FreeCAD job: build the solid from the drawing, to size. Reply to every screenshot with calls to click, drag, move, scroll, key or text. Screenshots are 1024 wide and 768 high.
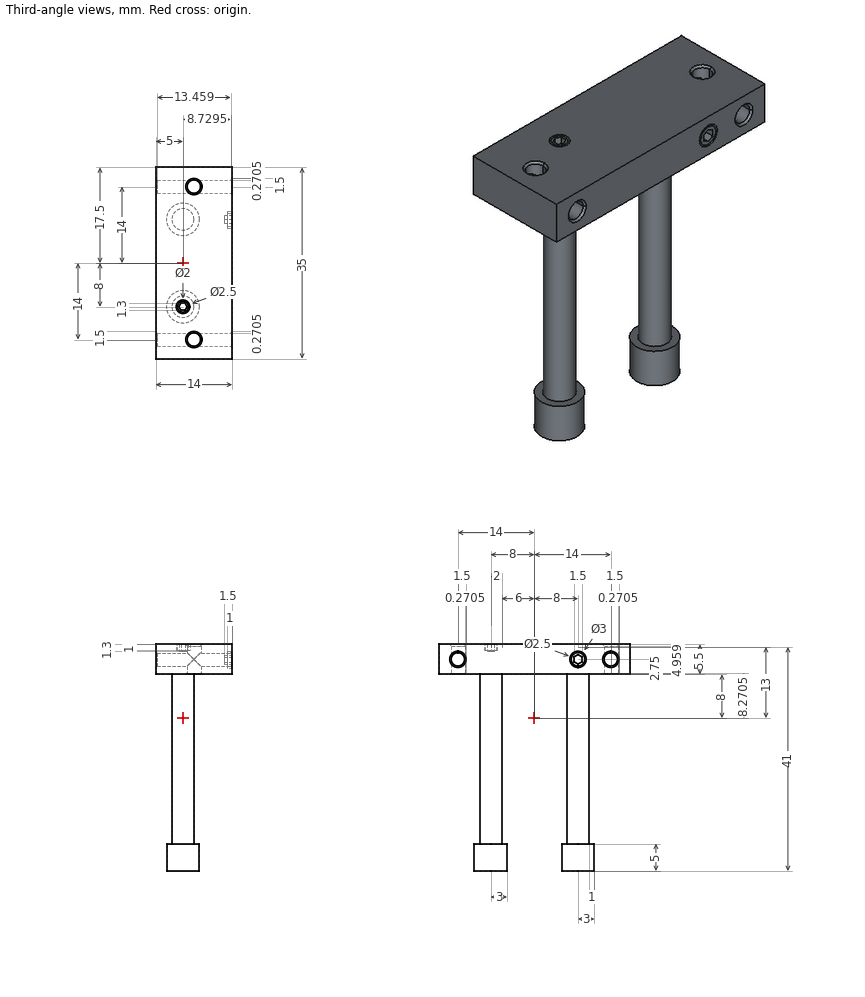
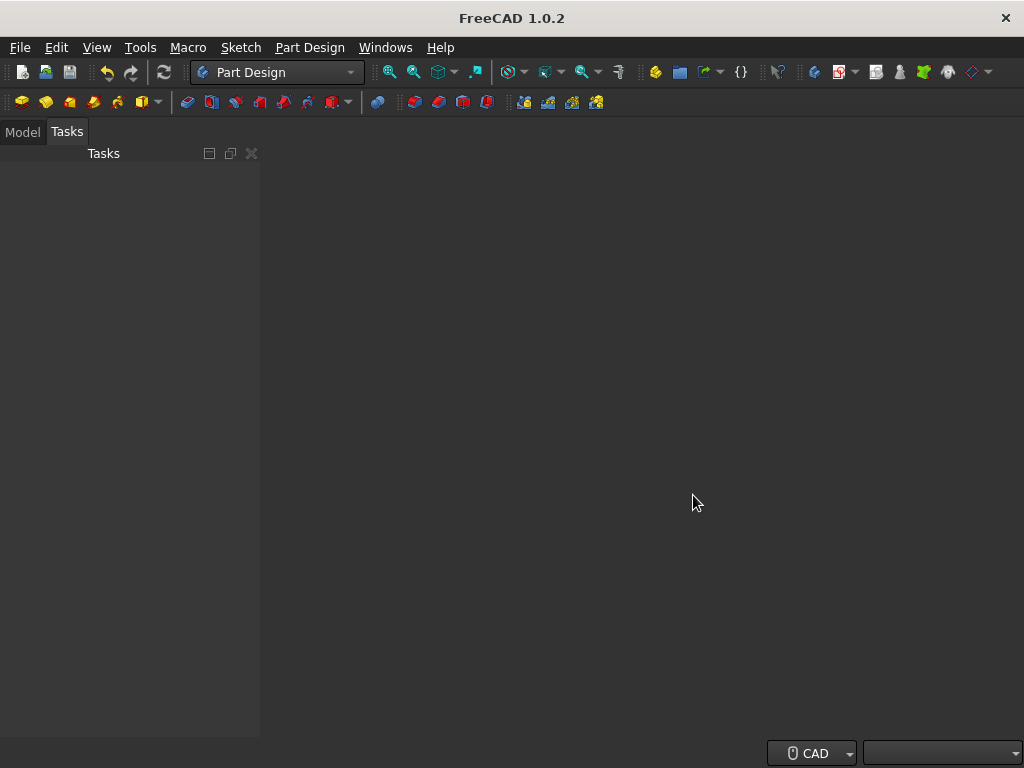
click(22, 72)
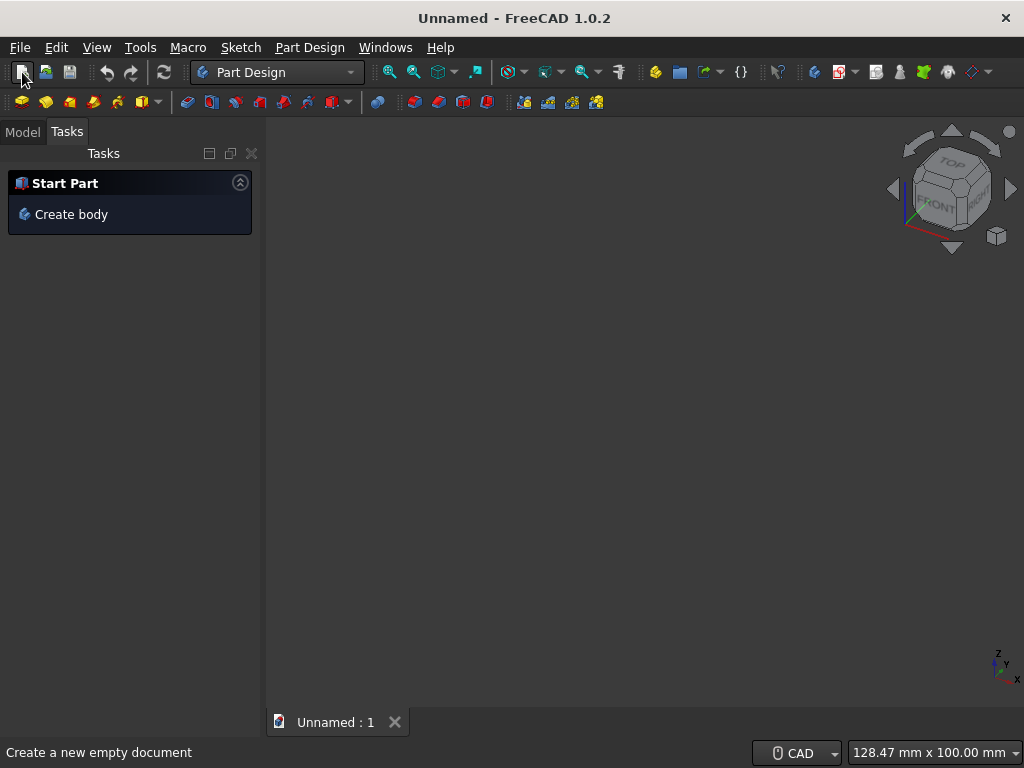
click(816, 72)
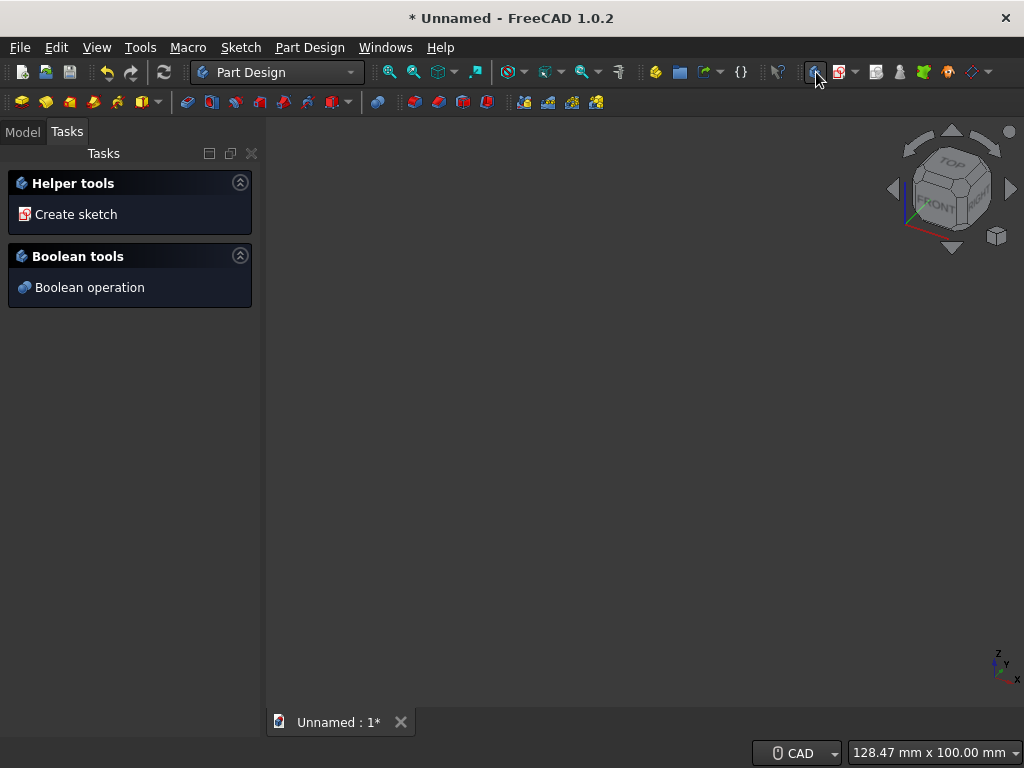
click(23, 131)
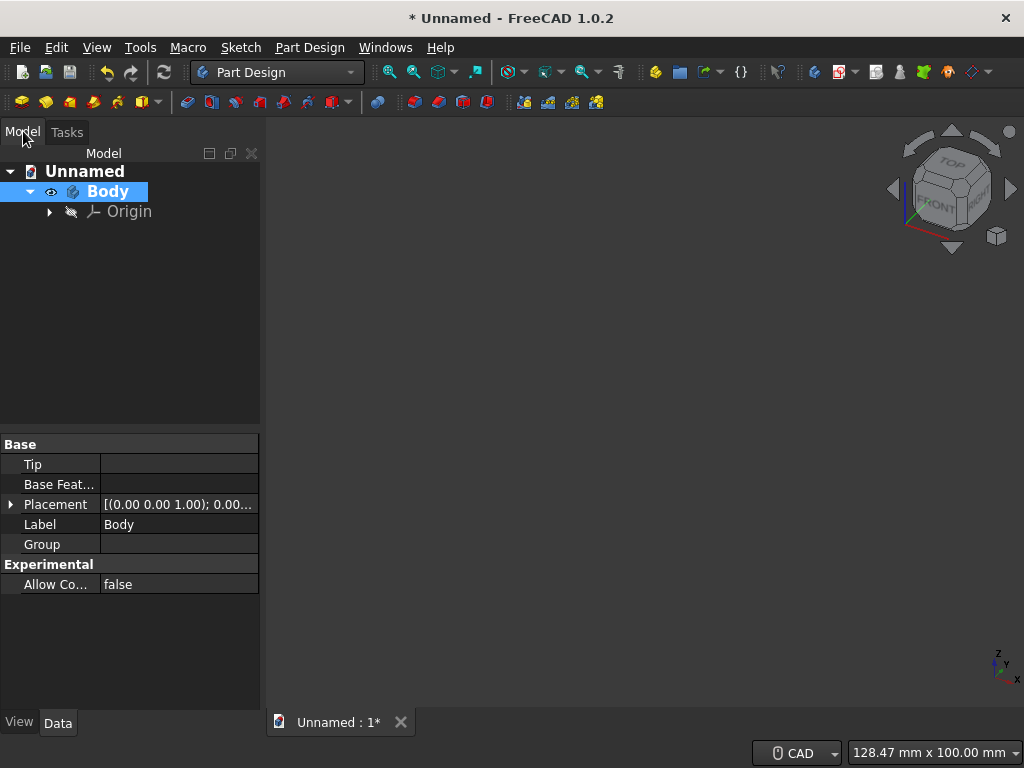
click(50, 212)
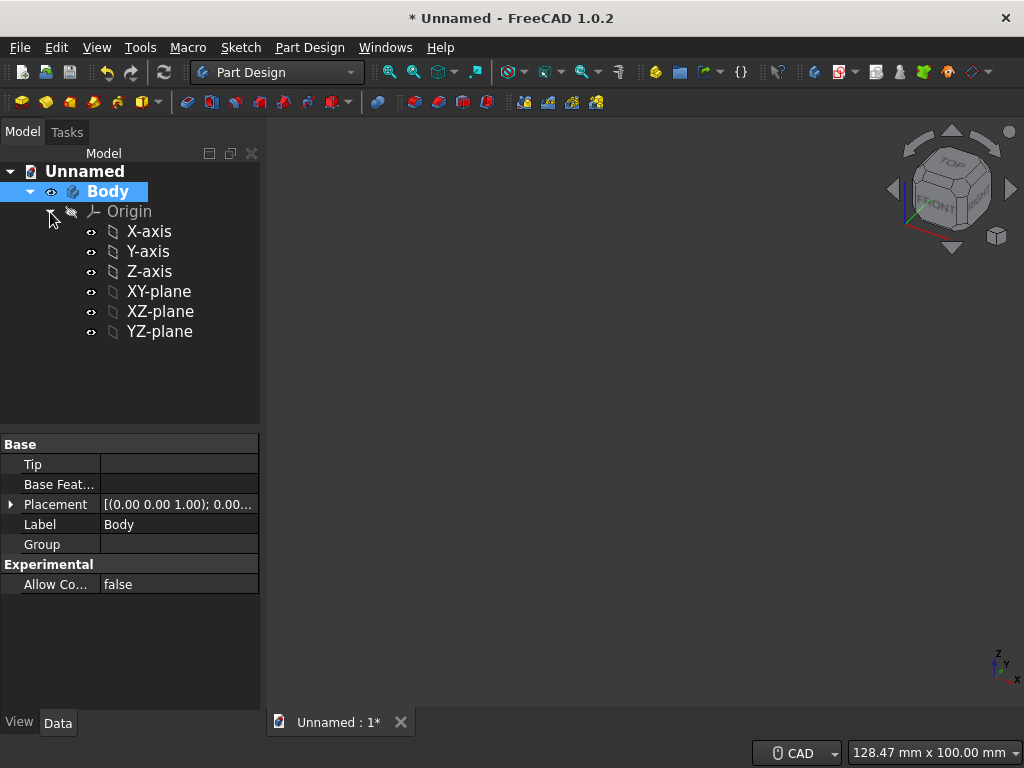
click(136, 292)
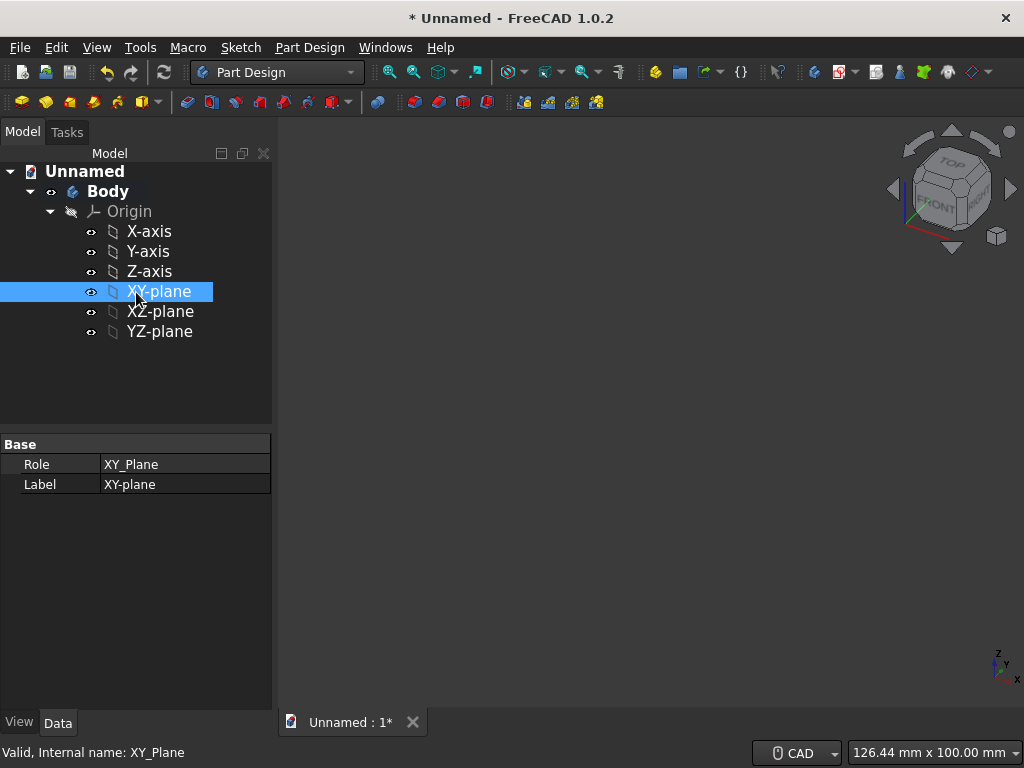
click(972, 72)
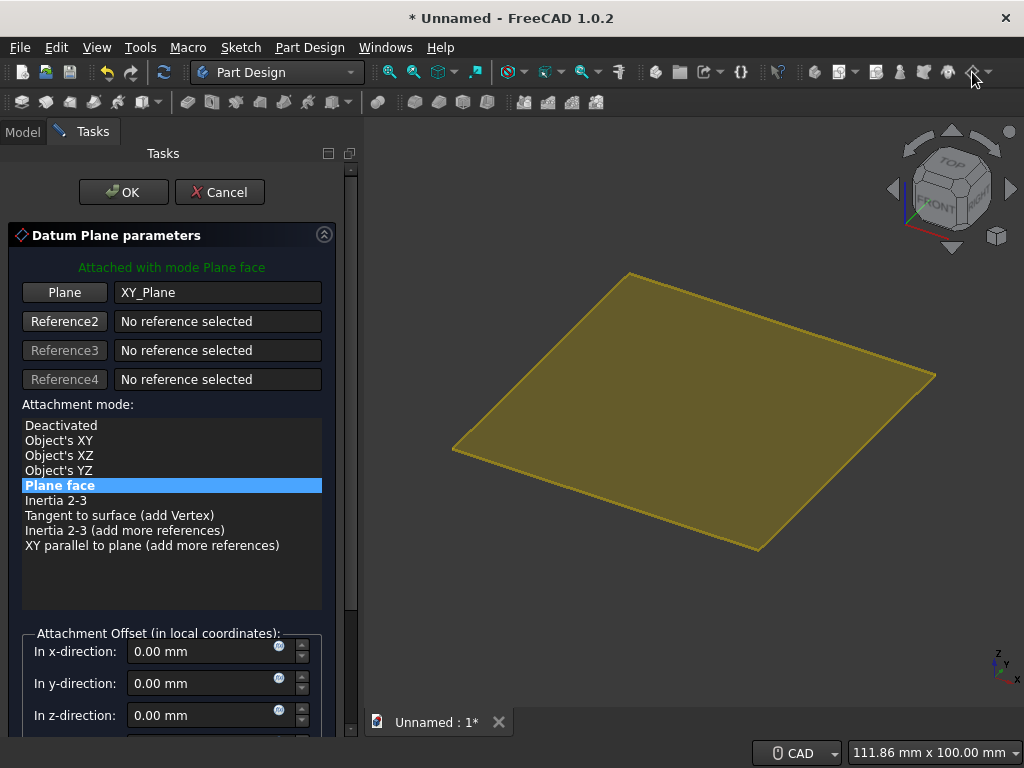
triple_click(210, 715)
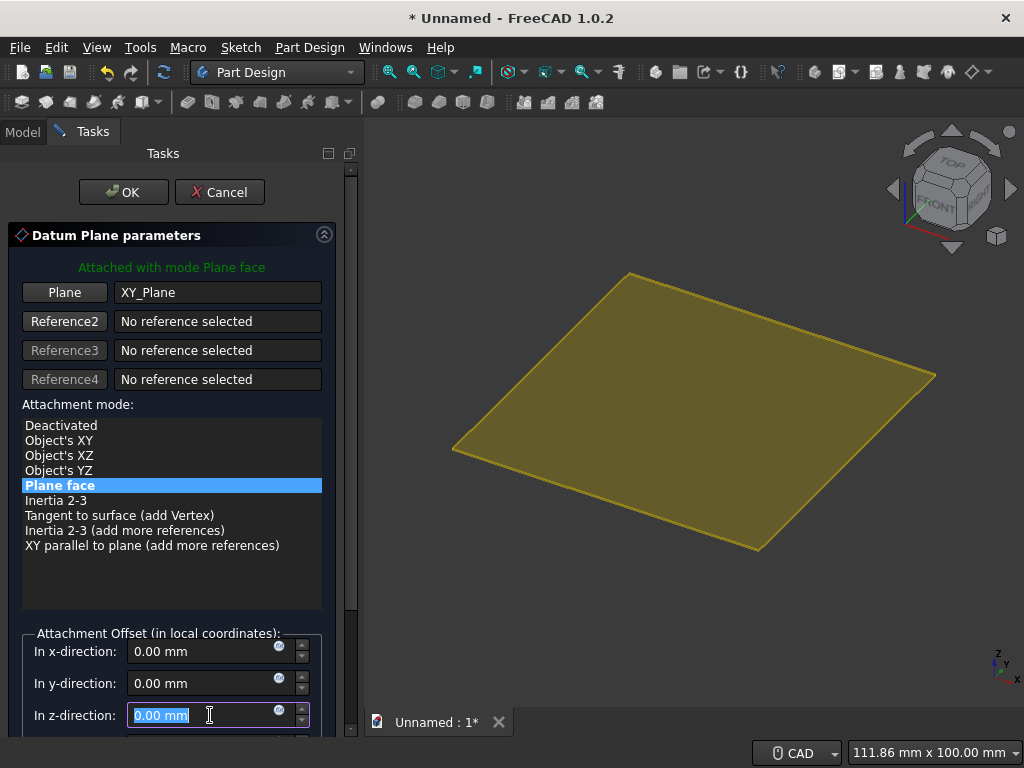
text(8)
key(Tab)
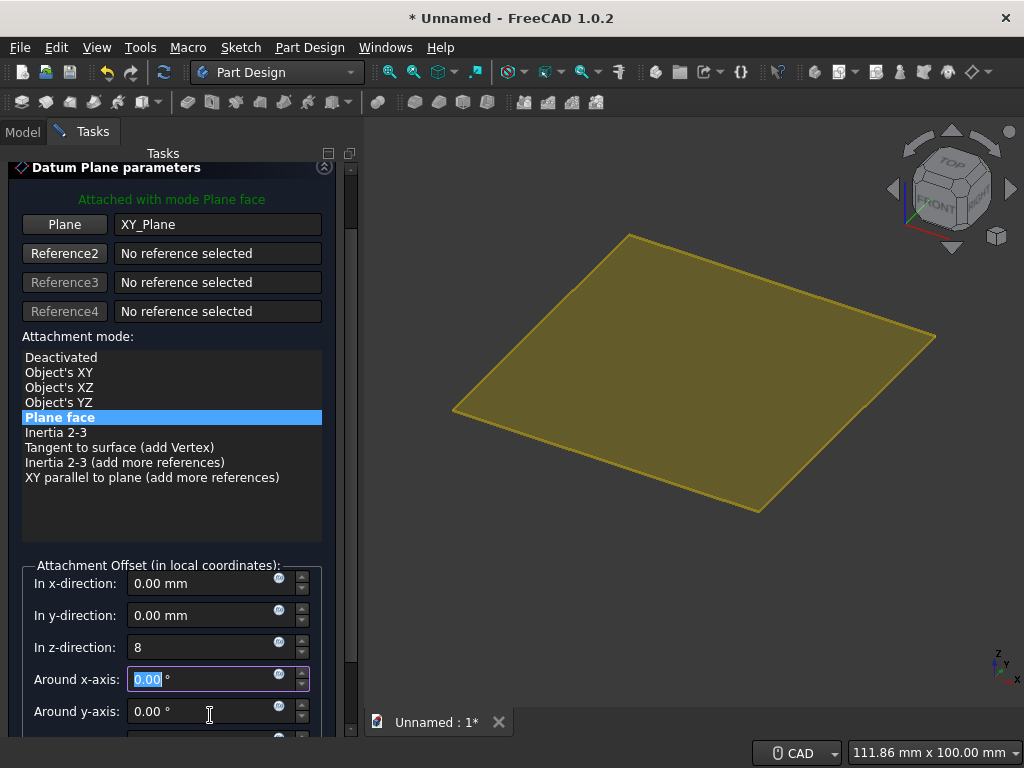
scroll(351, 450, up, 2)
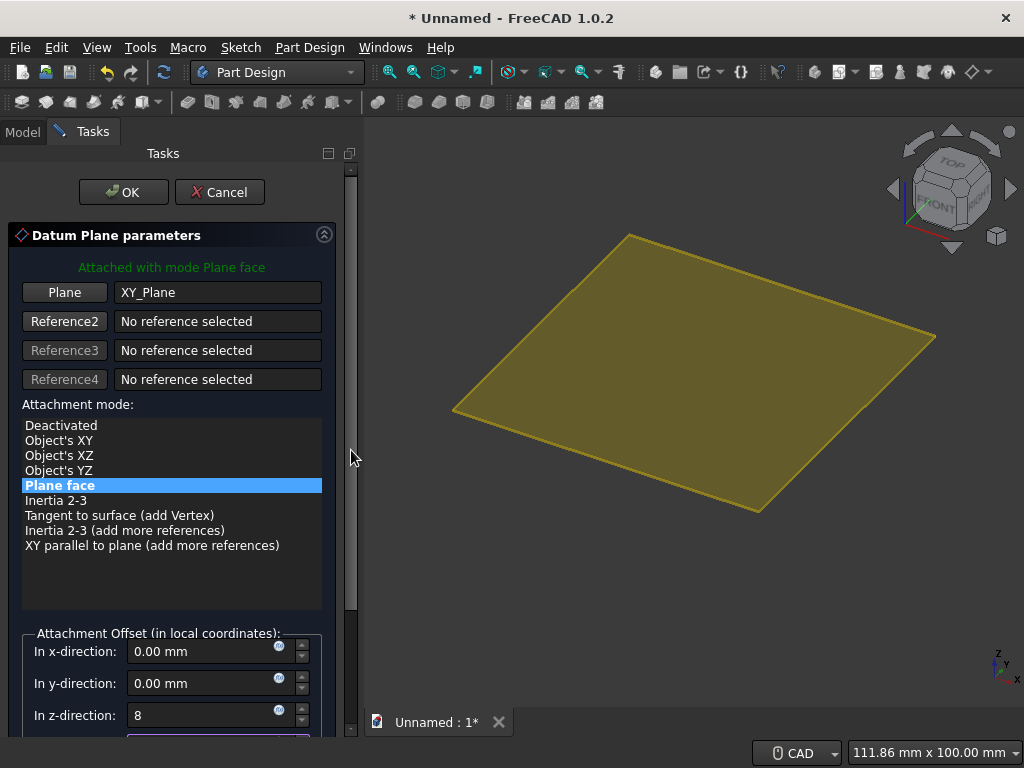
click(124, 192)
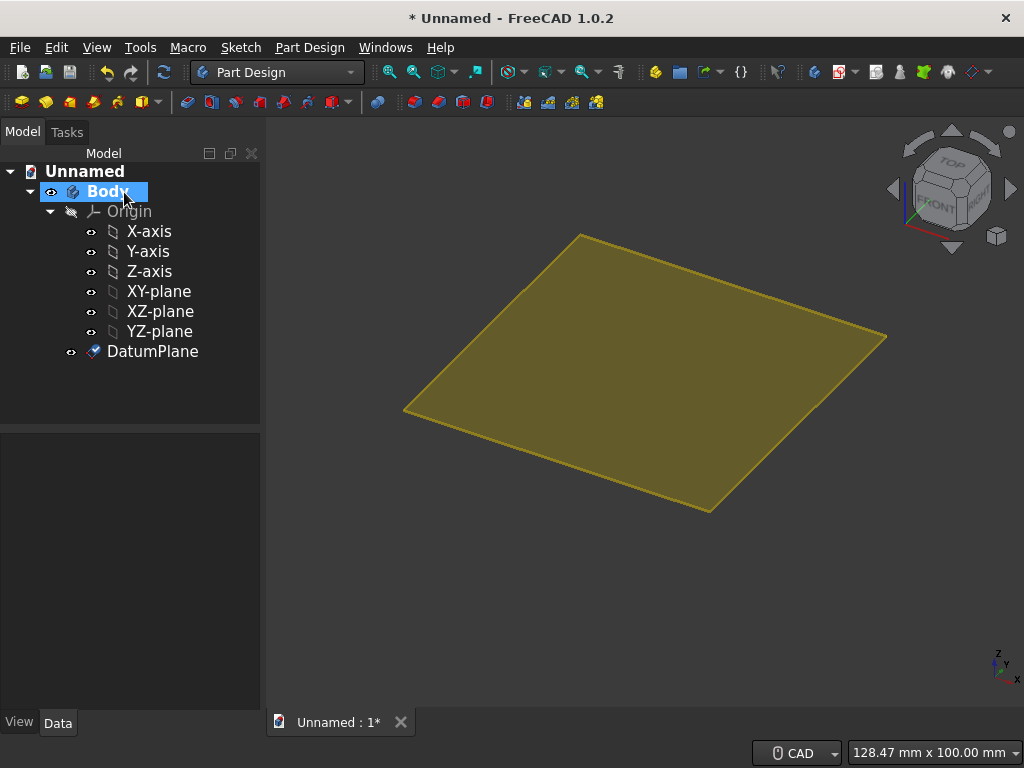
click(116, 352)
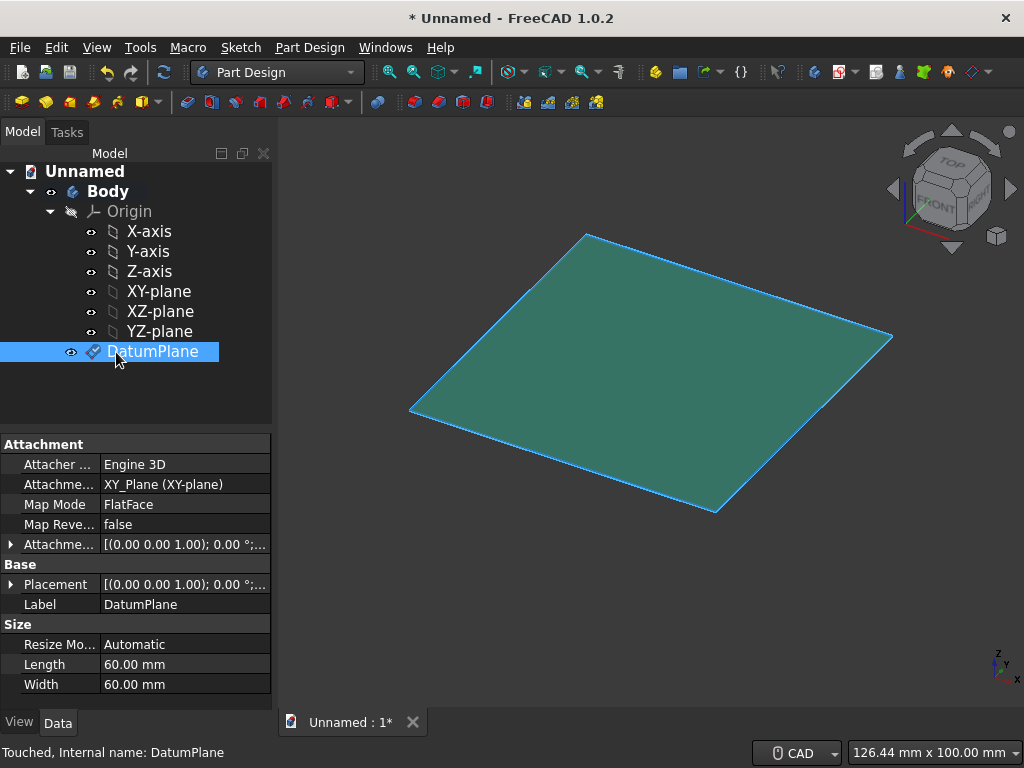
click(840, 72)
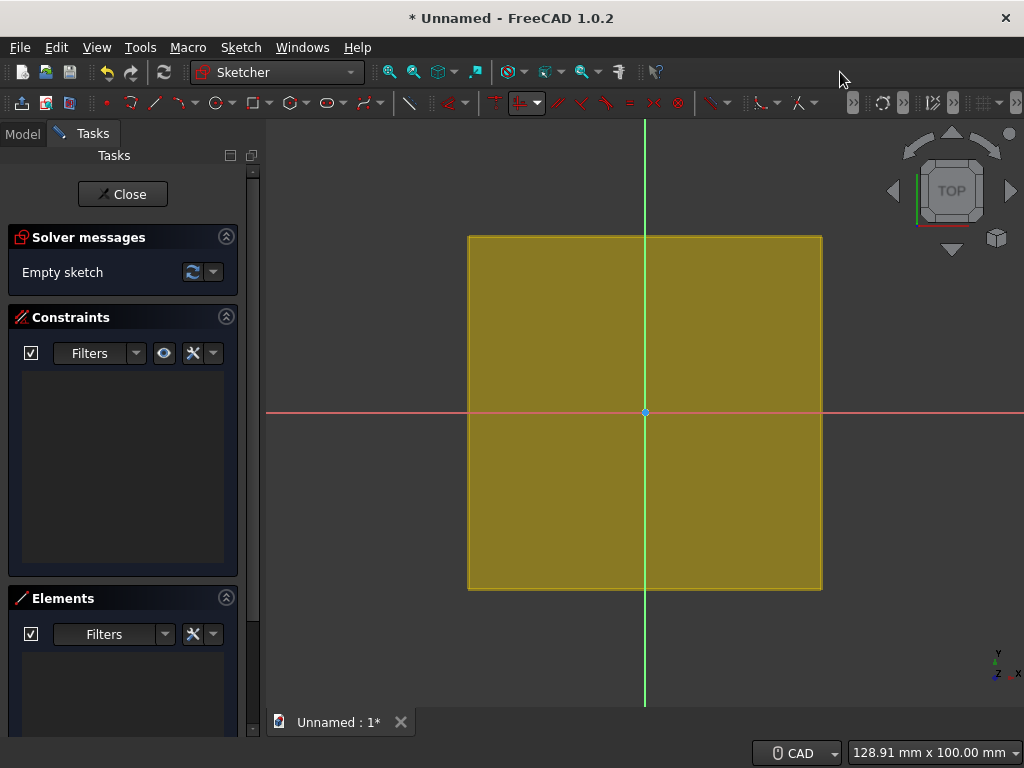
scroll(754, 413, up, 3)